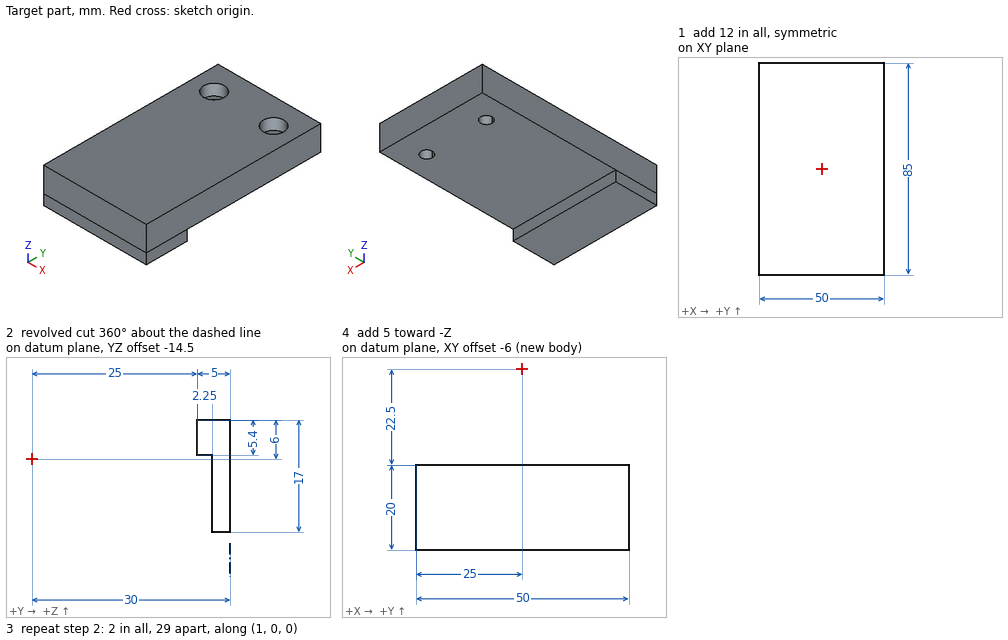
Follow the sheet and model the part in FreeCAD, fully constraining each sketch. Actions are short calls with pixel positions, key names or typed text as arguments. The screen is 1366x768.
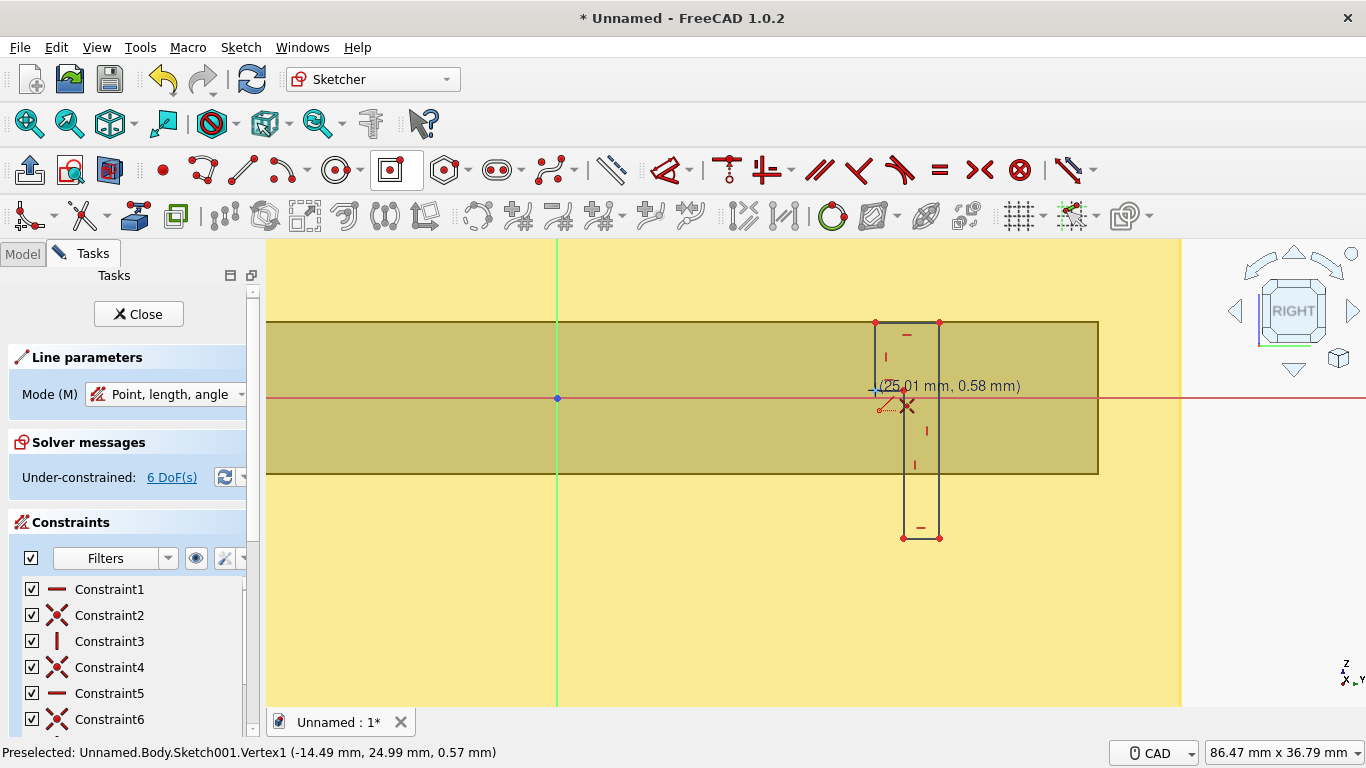
click(939, 560)
click(939, 624)
key(Escape)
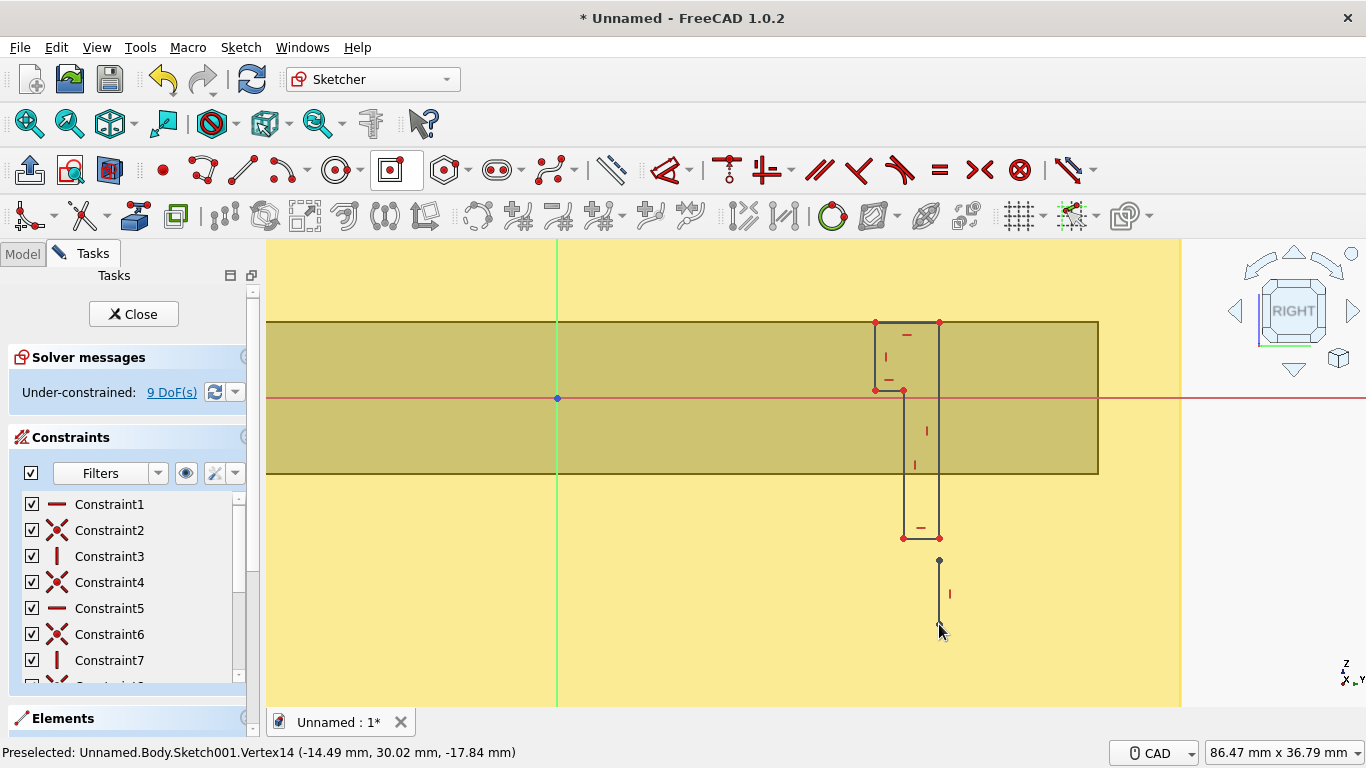
click(939, 580)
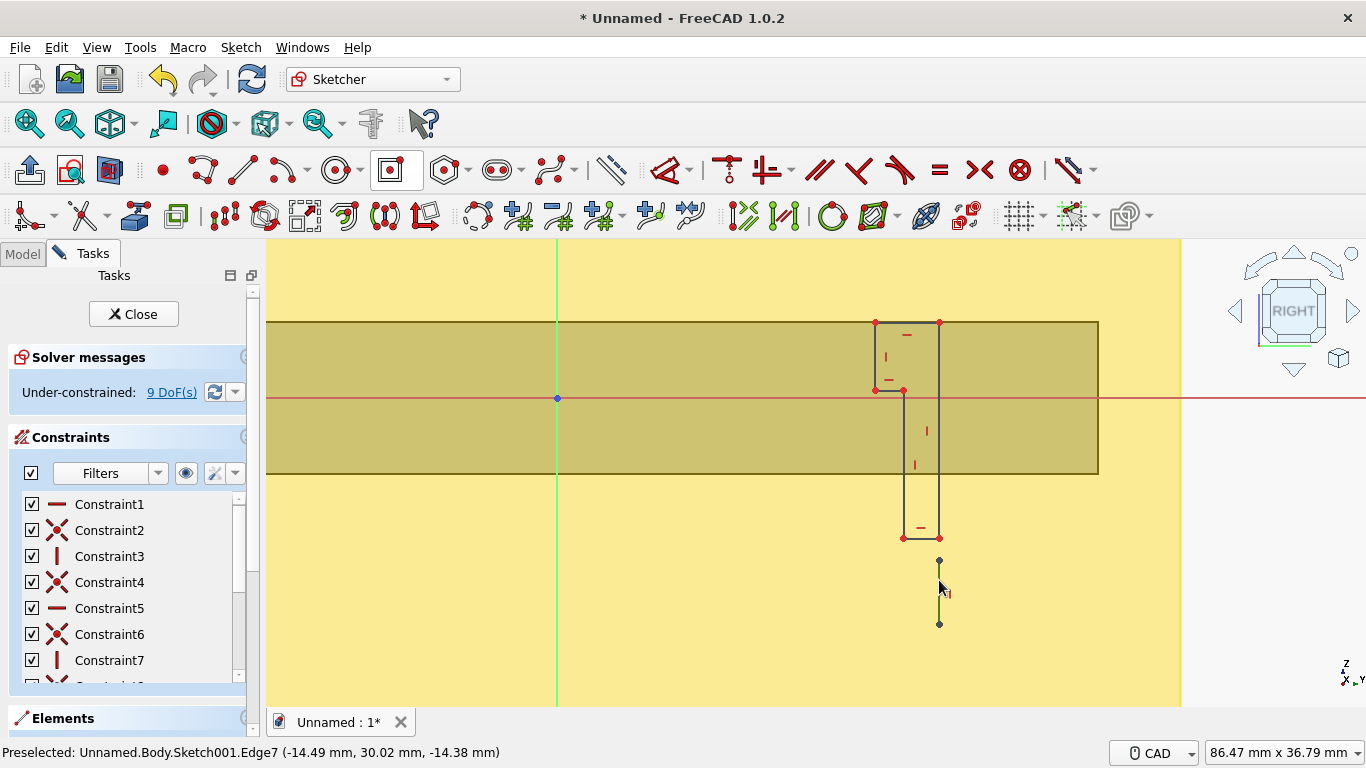
key(g)
key(n)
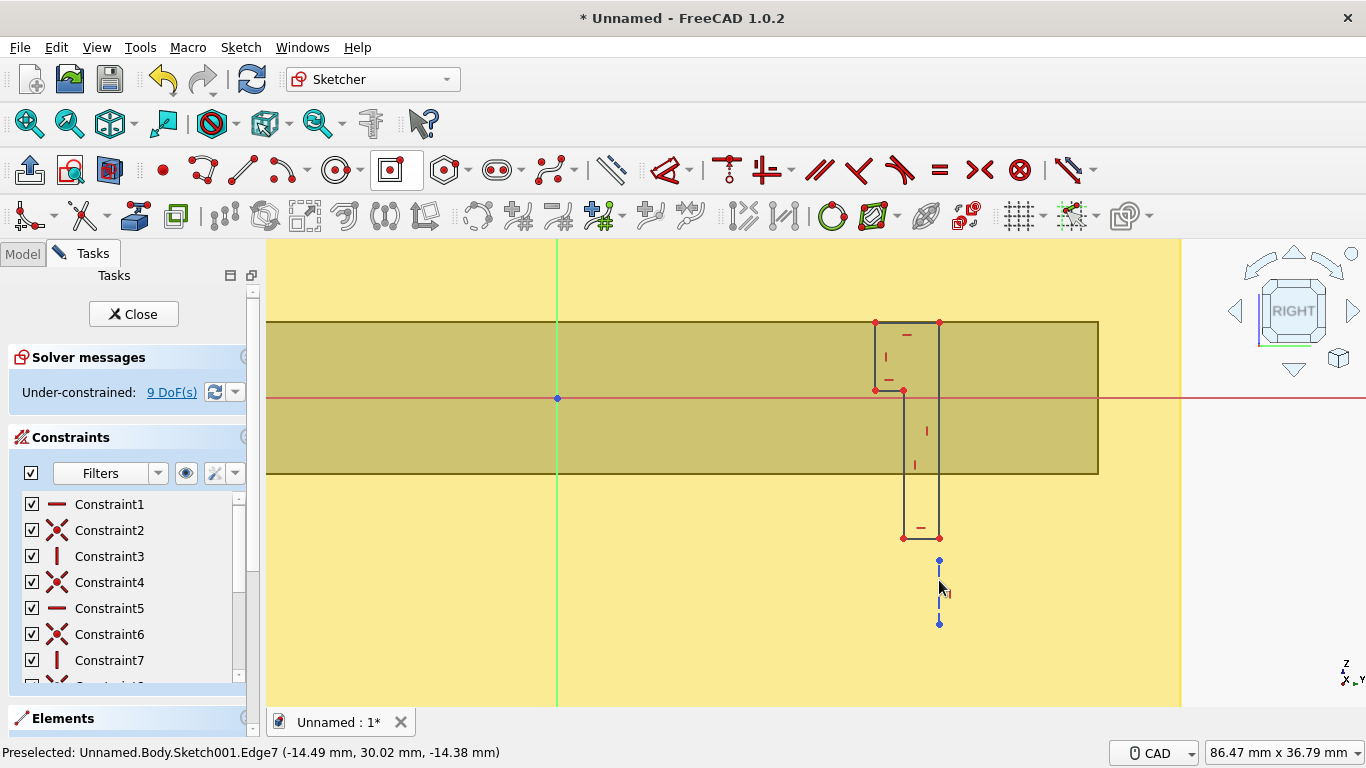
key(d)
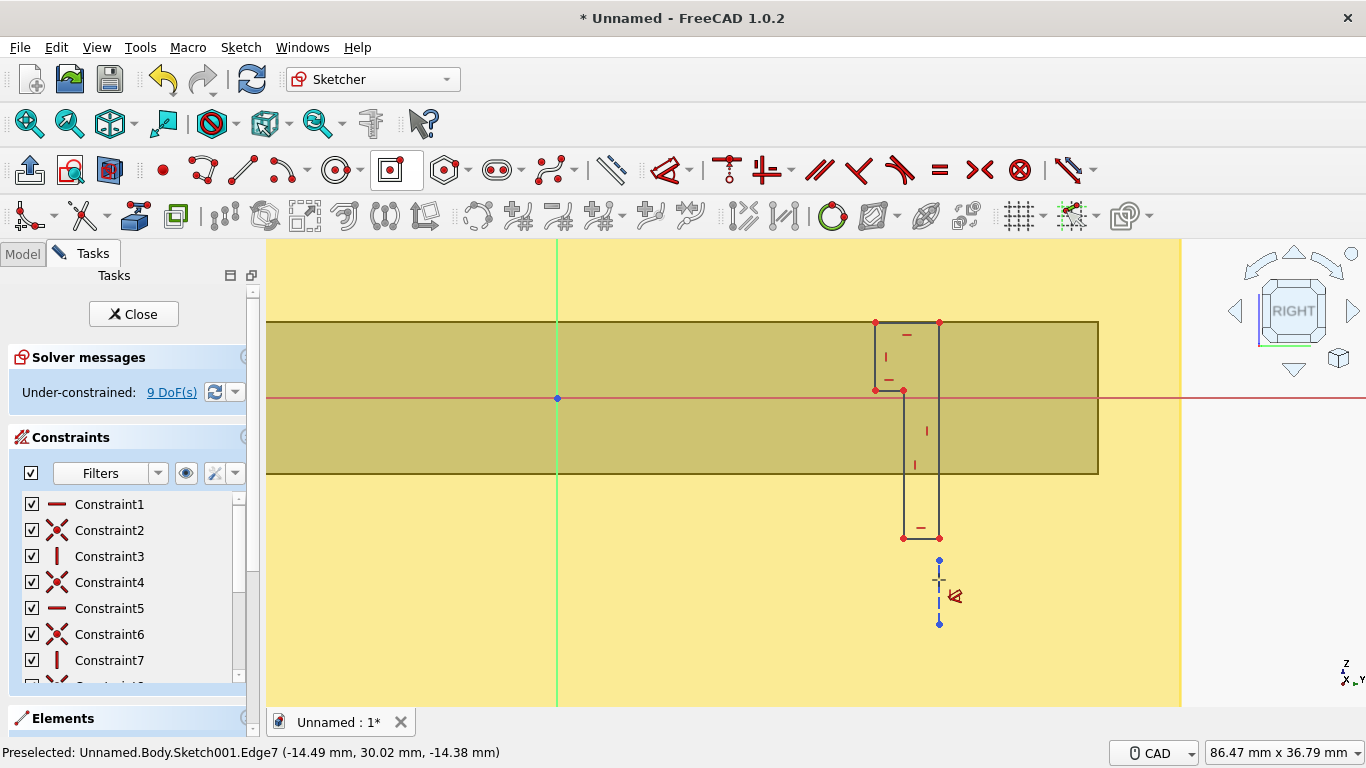
click(920, 323)
click(907, 289)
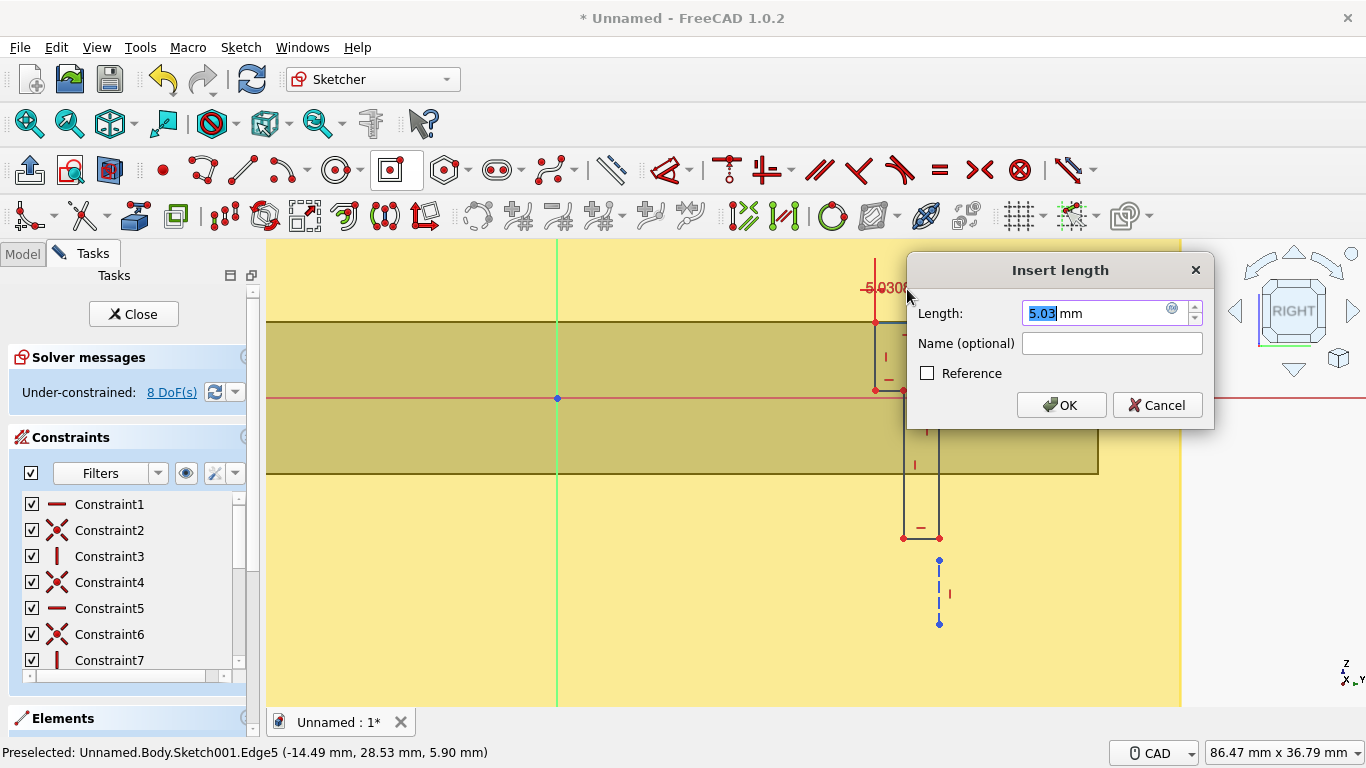
text(5)
key(Return)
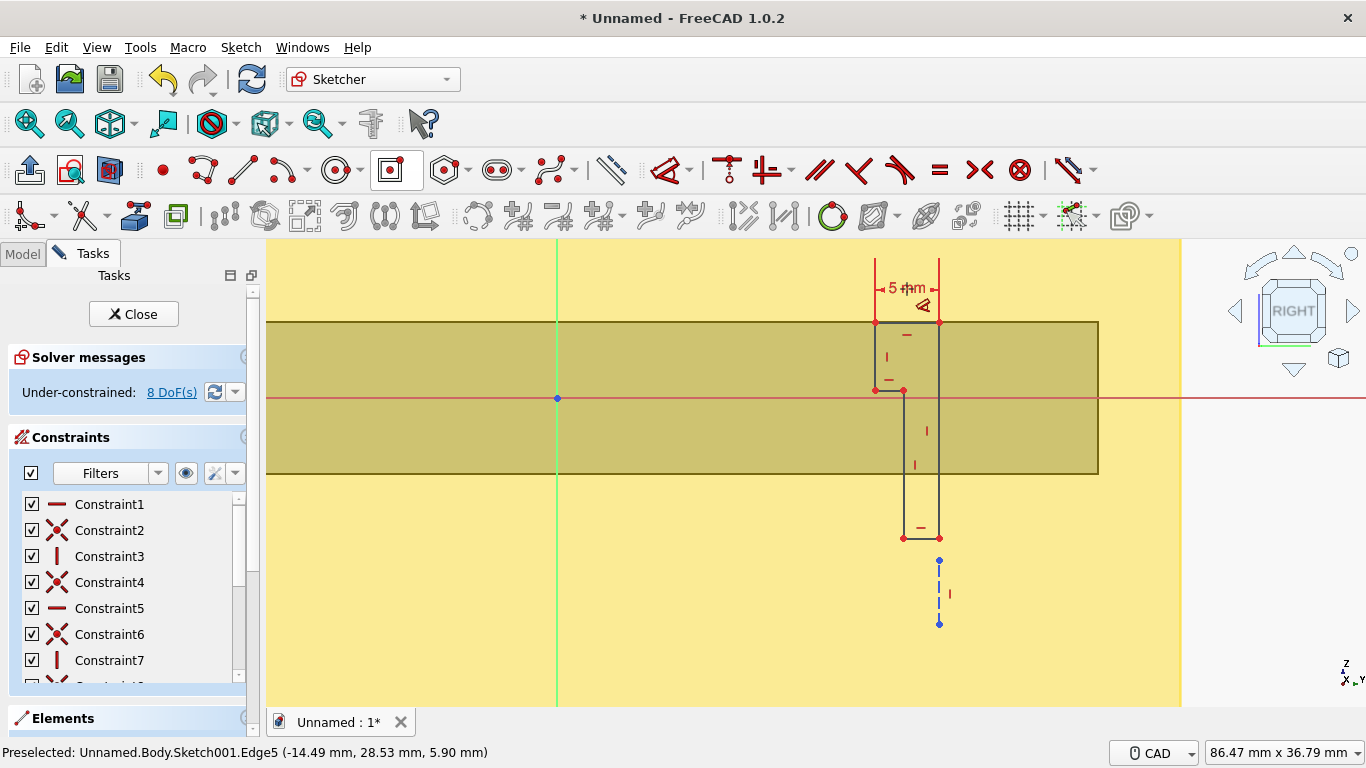
click(939, 474)
click(973, 431)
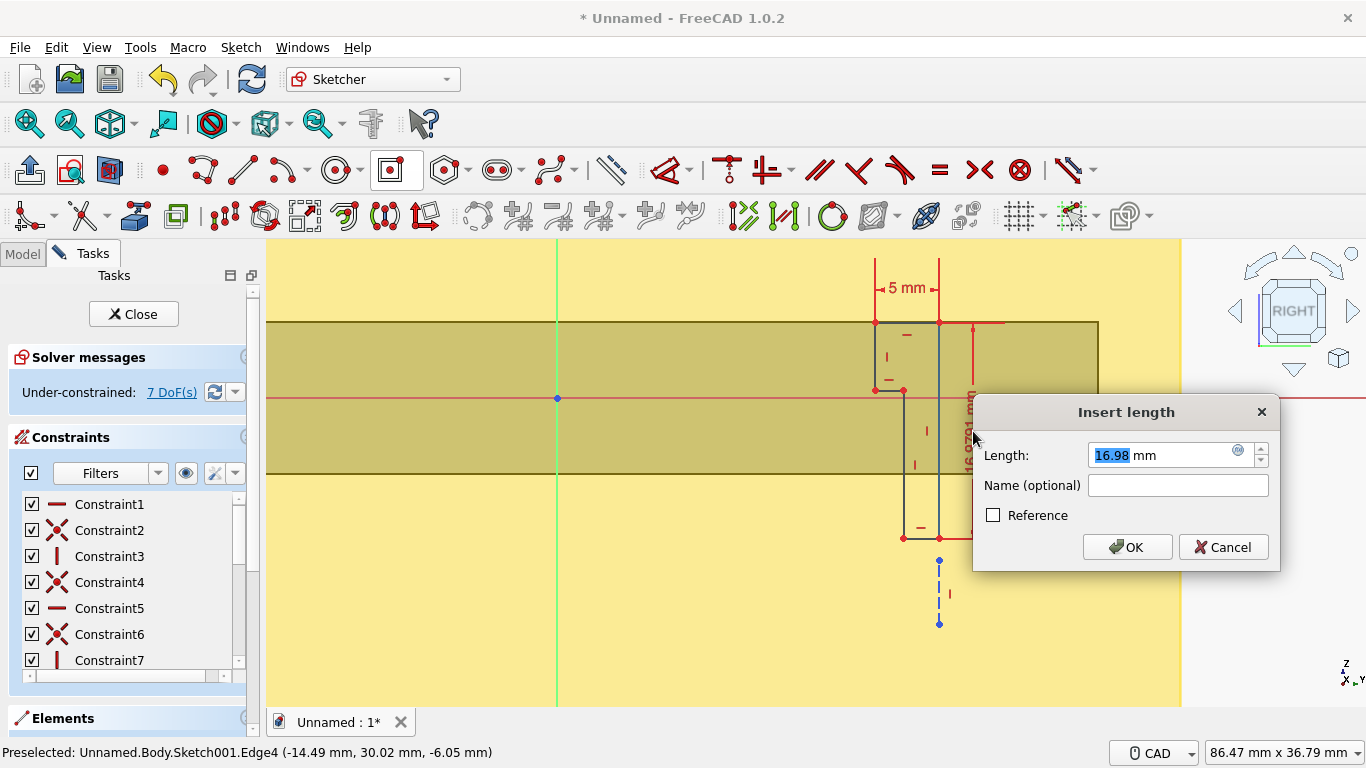
text(17)
key(Return)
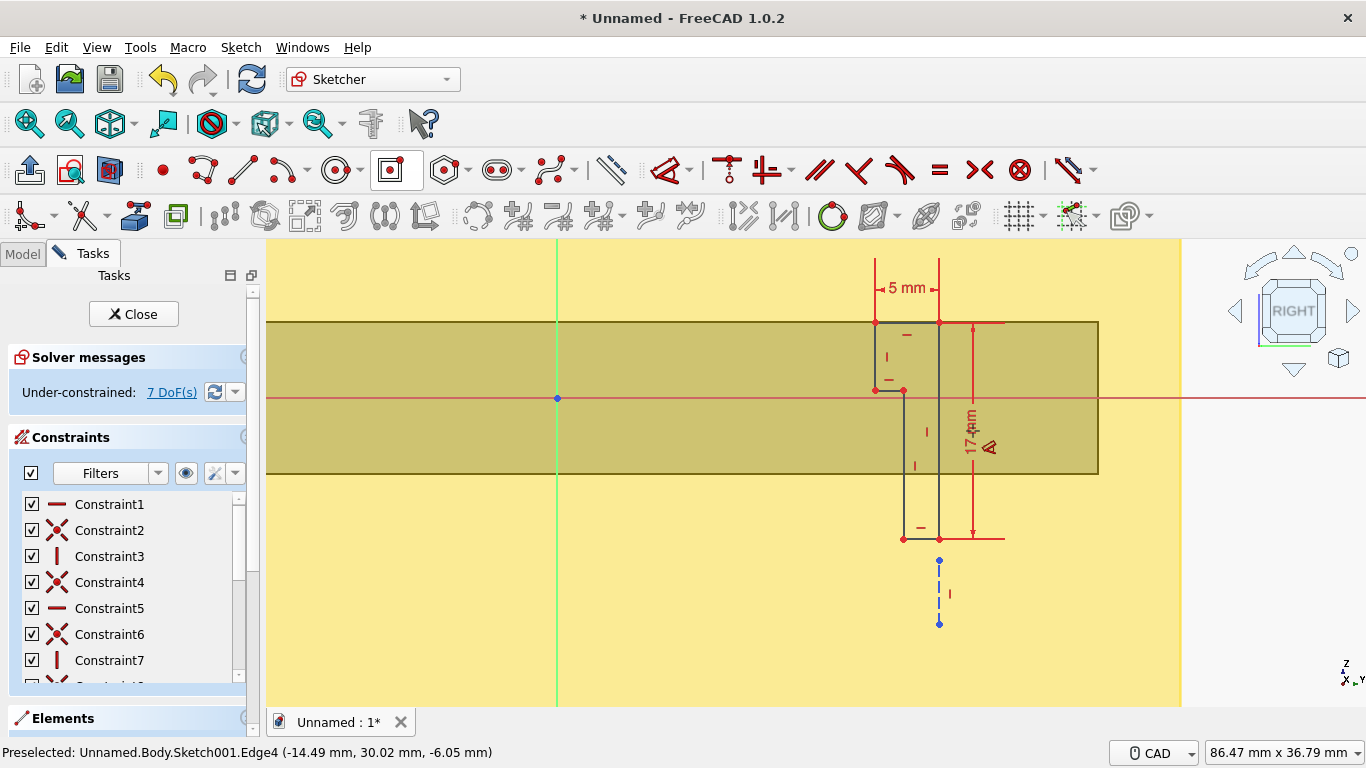
click(939, 323)
click(973, 361)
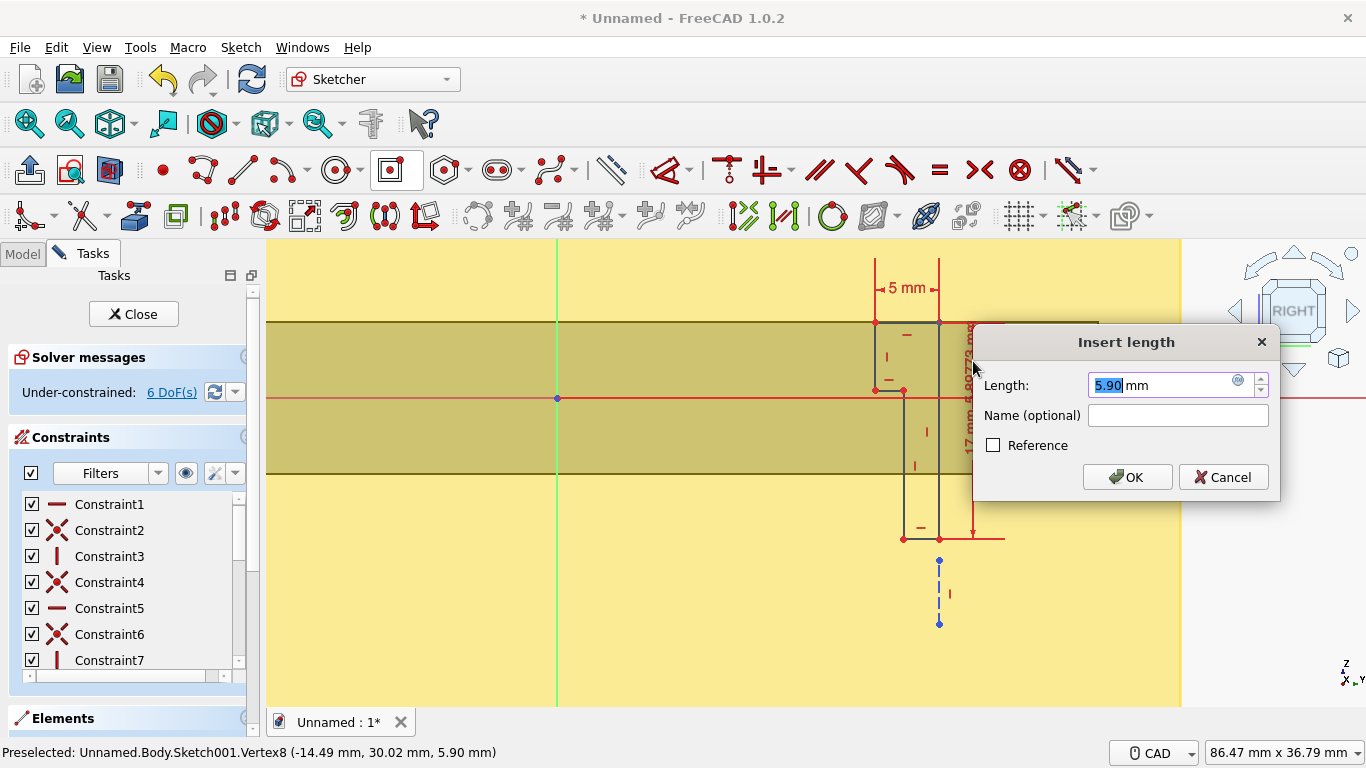
text(6)
key(Return)